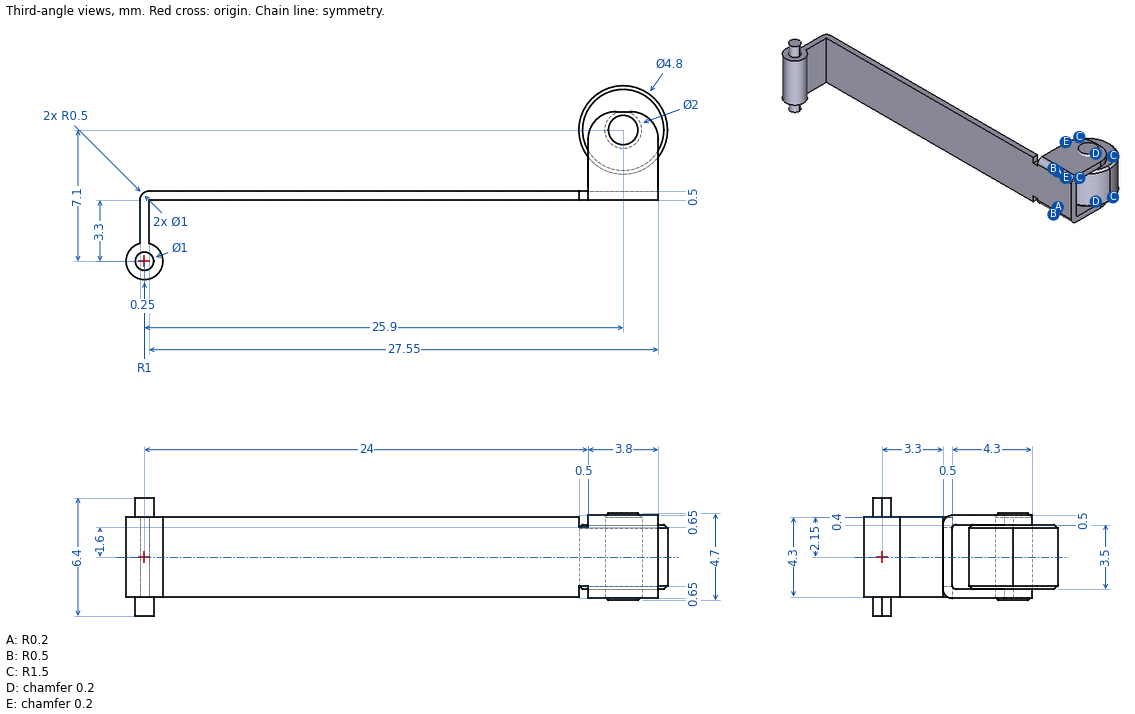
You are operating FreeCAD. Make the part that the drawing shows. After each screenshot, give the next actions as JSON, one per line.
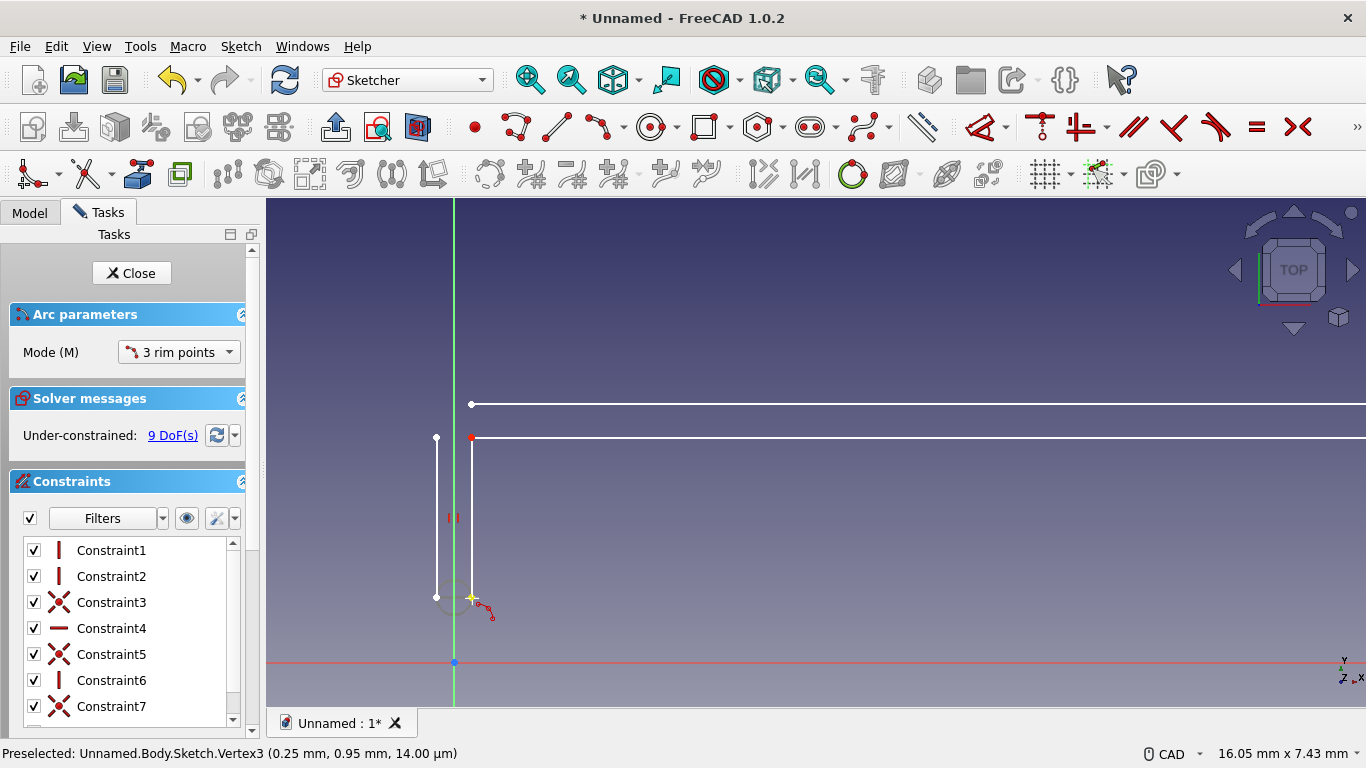
{"action": "scroll", "coordinate": [471, 403], "scroll_direction": "down", "scroll_amount": 6}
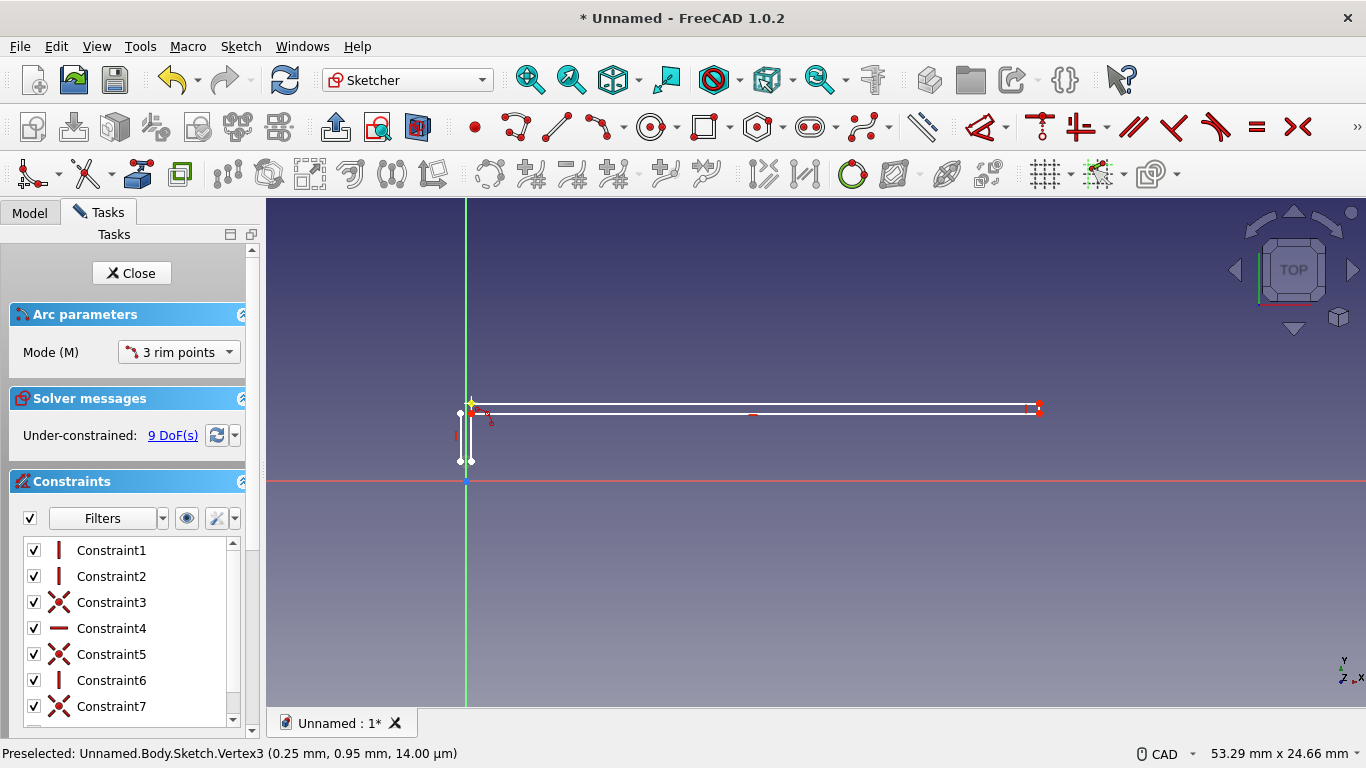
{"action": "scroll", "coordinate": [455, 499], "scroll_direction": "up", "scroll_amount": 2}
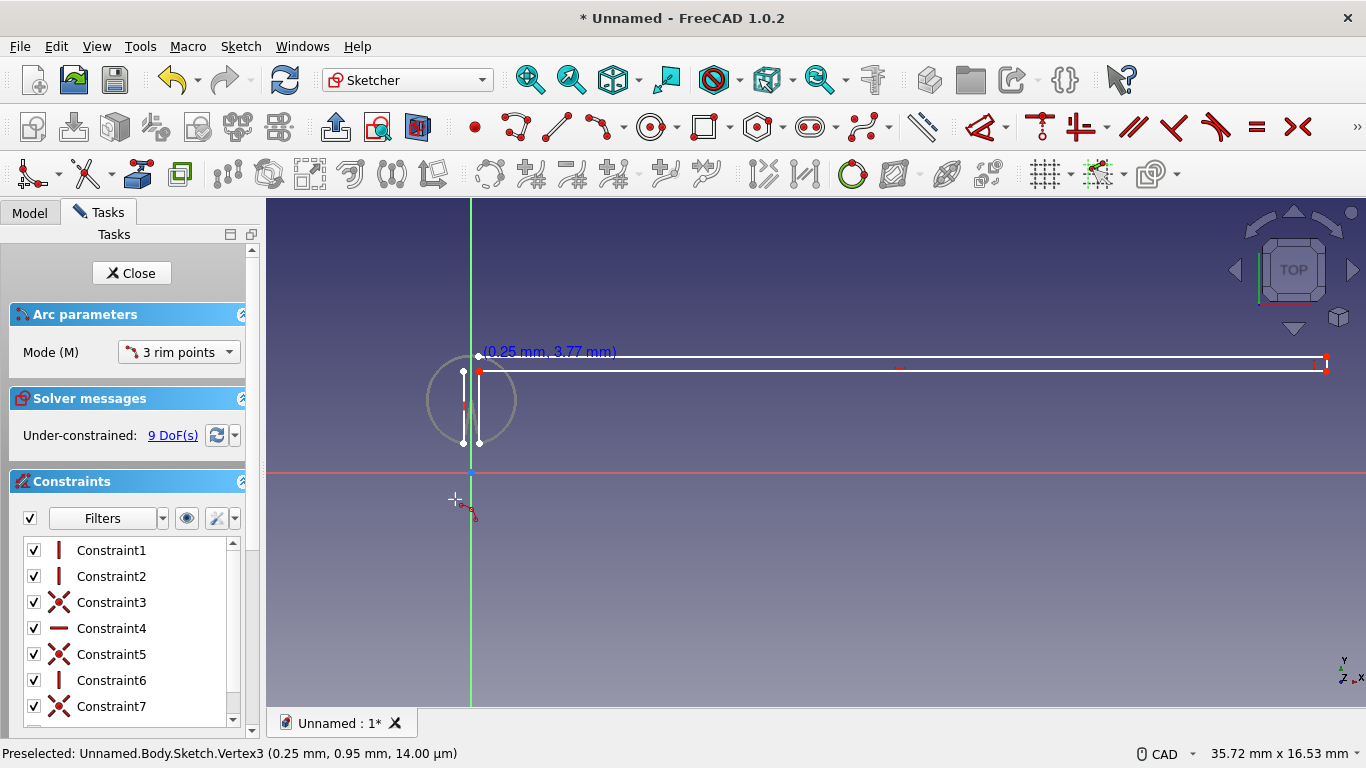
{"action": "left_click", "coordinate": [455, 498]}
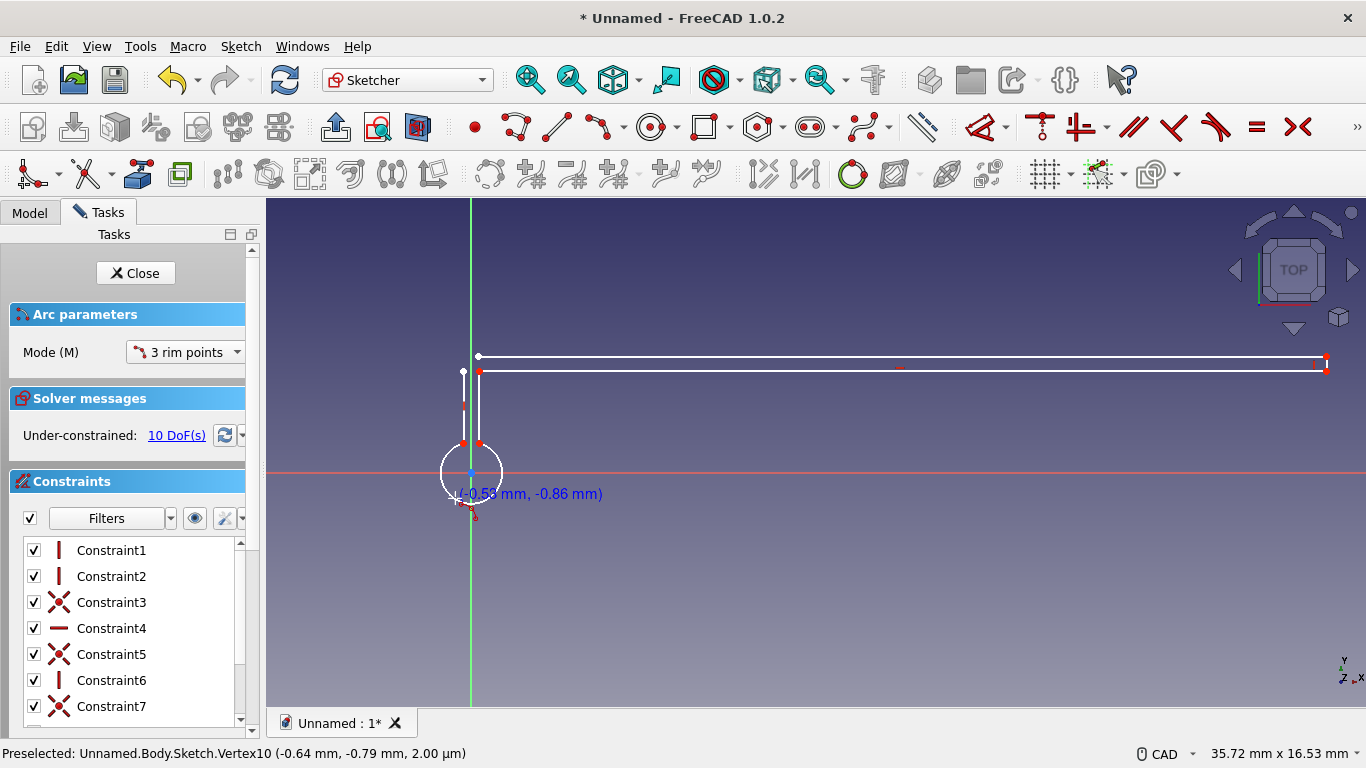
{"action": "scroll", "coordinate": [479, 356], "scroll_direction": "up", "scroll_amount": 4}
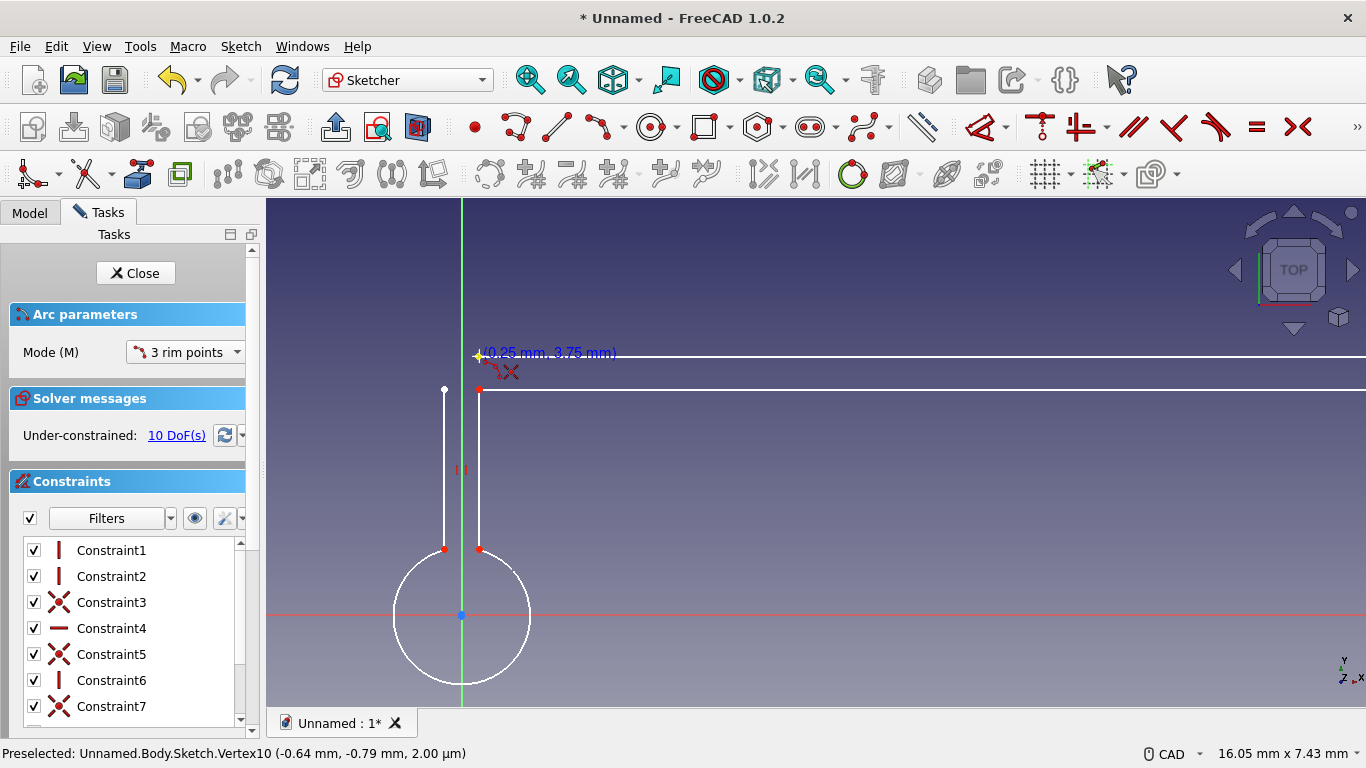
{"action": "left_click", "coordinate": [479, 357]}
{"action": "left_click", "coordinate": [444, 390]}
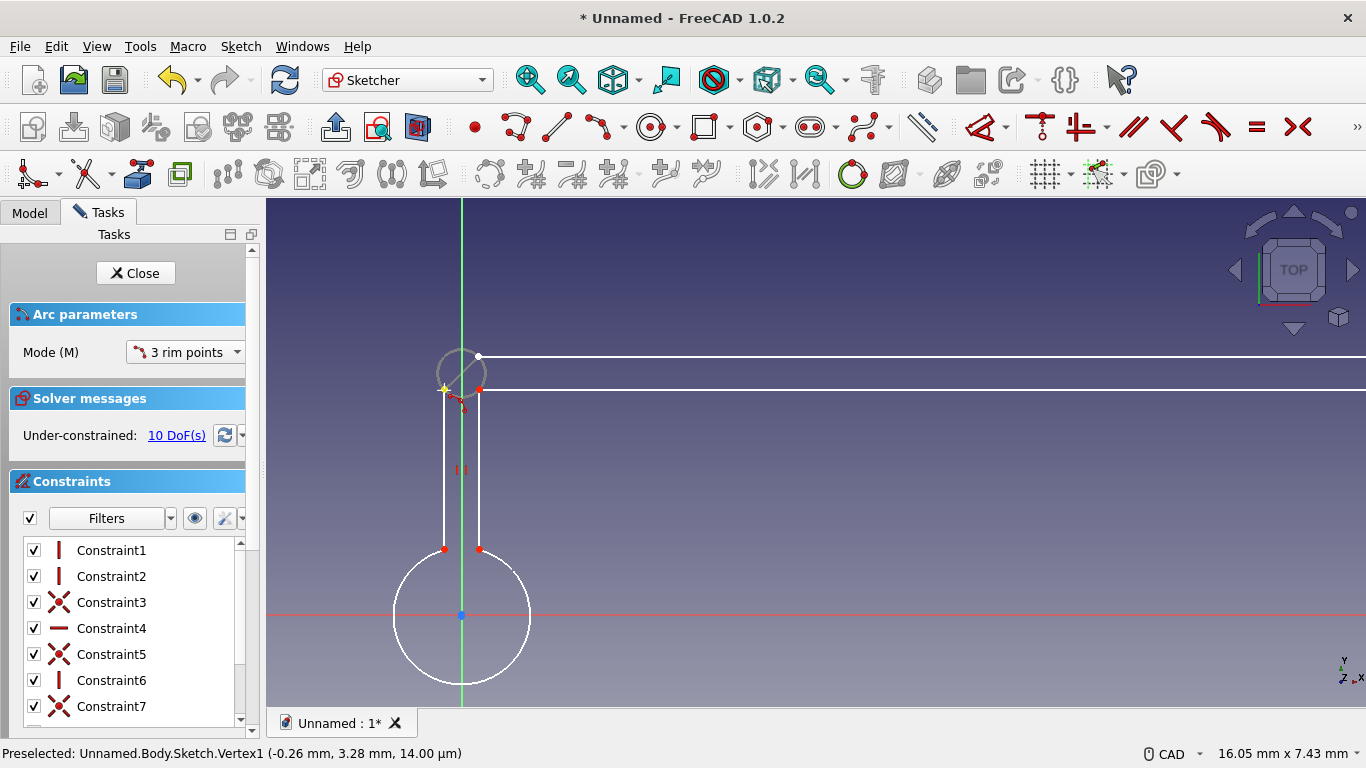
{"action": "scroll", "coordinate": [451, 369], "scroll_direction": "up", "scroll_amount": 3}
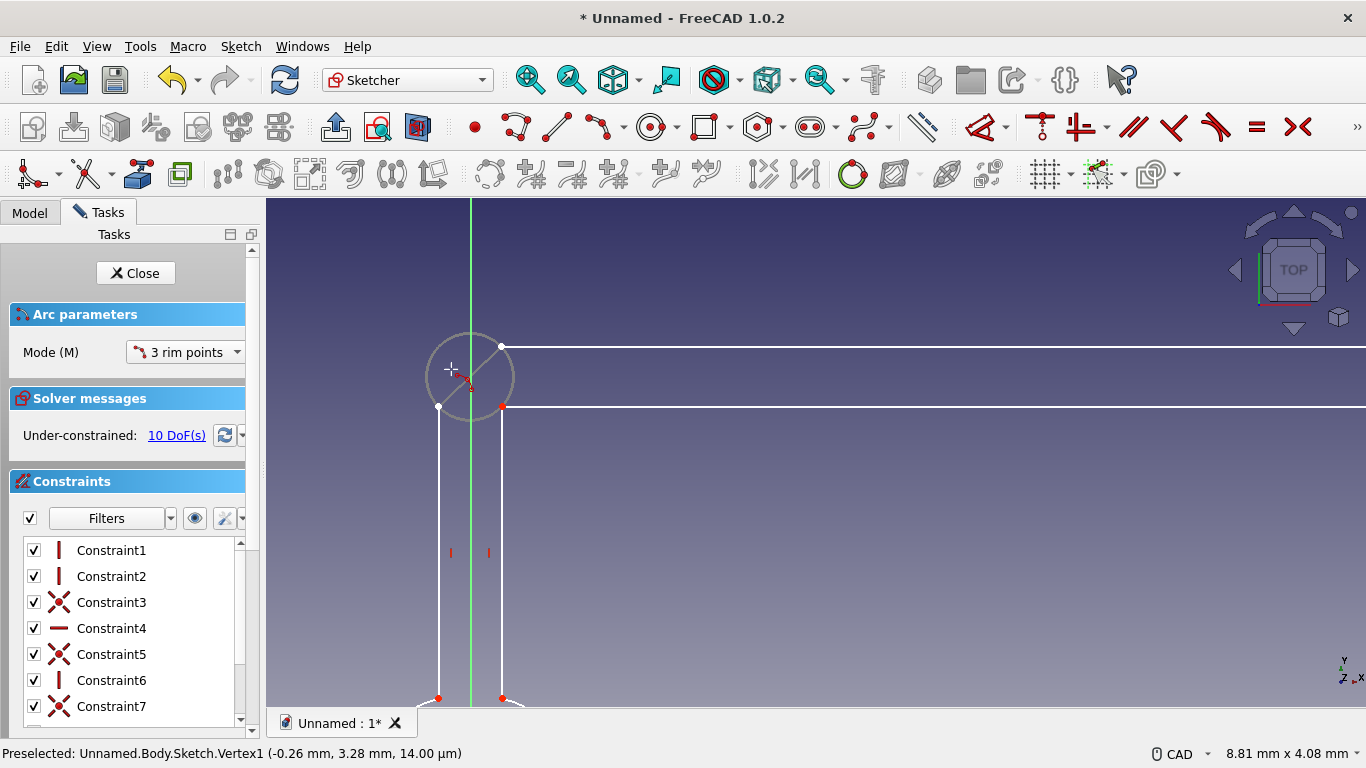
{"action": "left_click", "coordinate": [451, 368]}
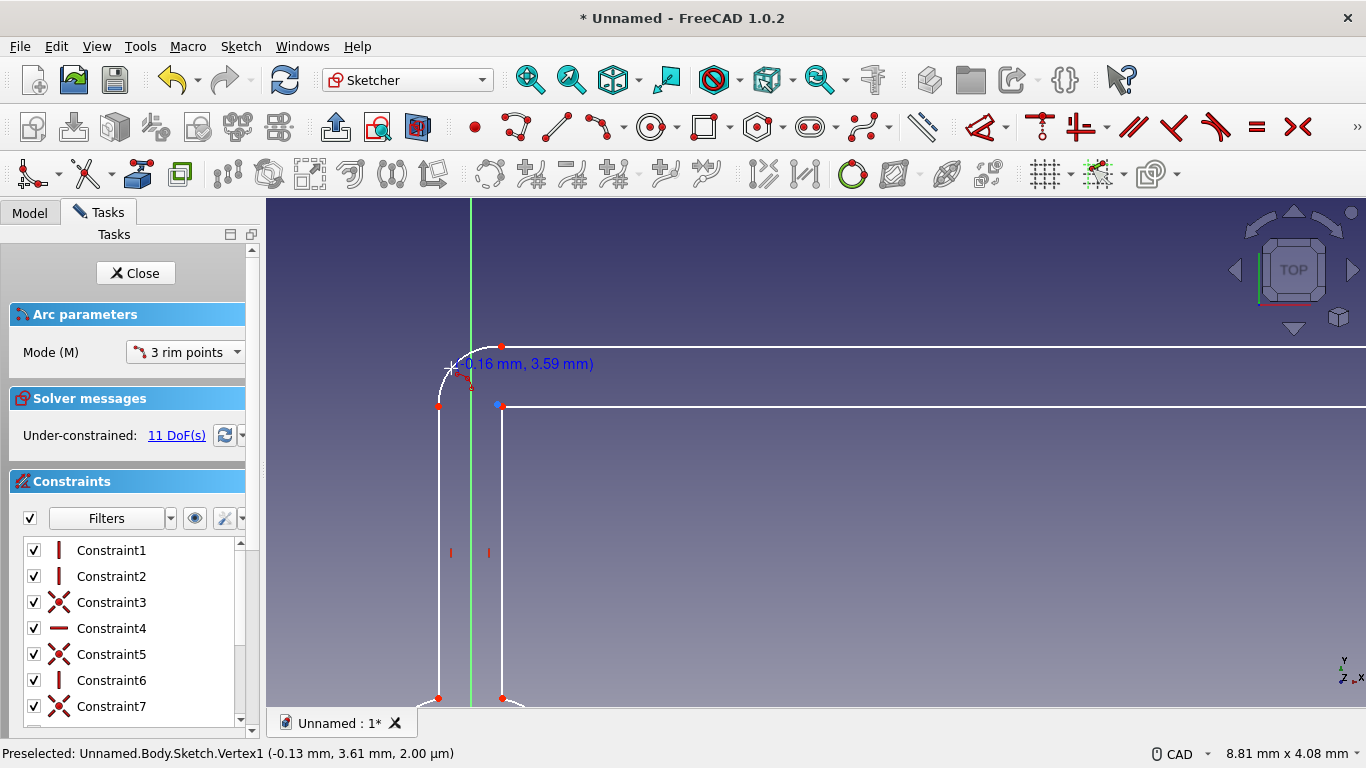
{"action": "left_click", "coordinate": [650, 128]}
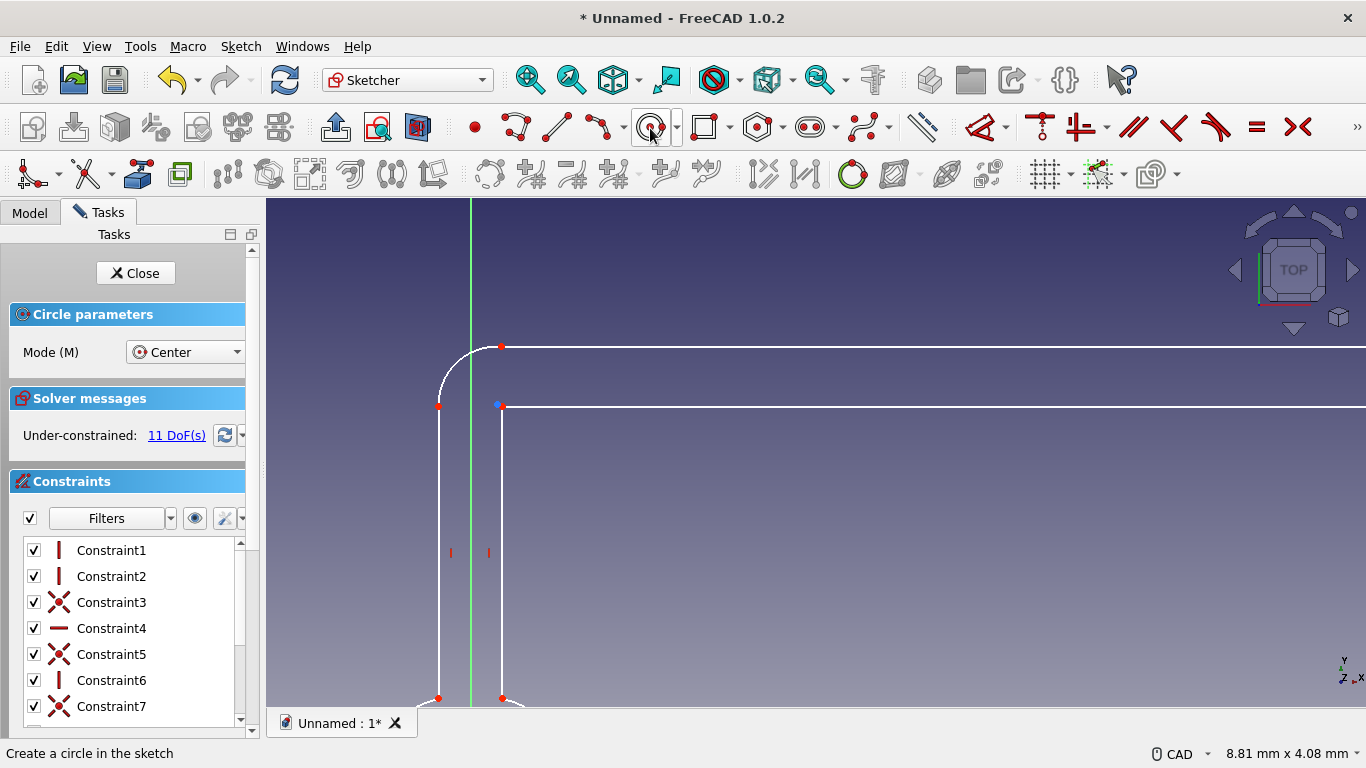
{"action": "scroll", "coordinate": [465, 415], "scroll_direction": "down", "scroll_amount": 9}